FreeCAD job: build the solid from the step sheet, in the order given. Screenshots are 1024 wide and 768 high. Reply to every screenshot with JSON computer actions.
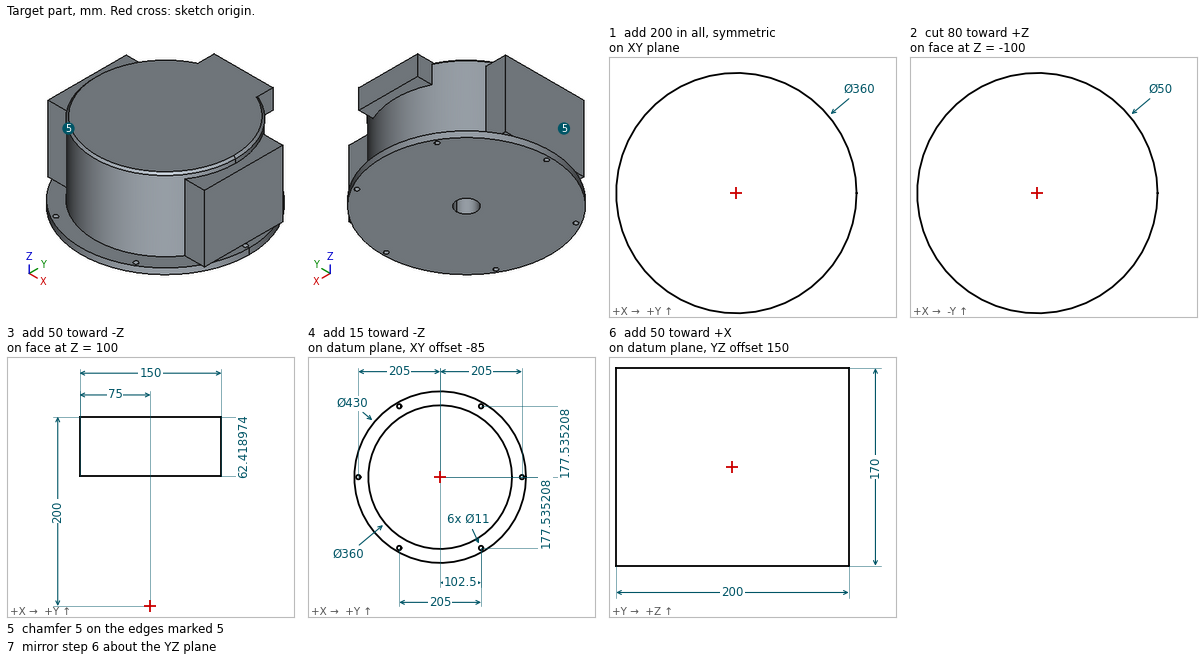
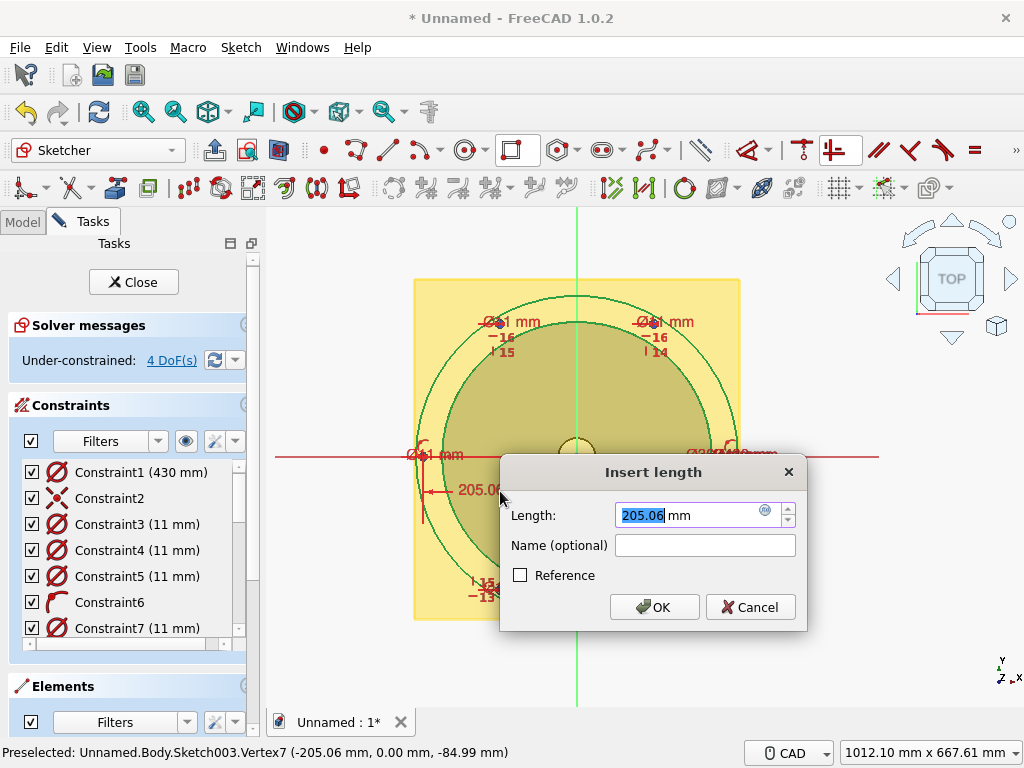
{"action": "type", "text": "205"}
{"action": "key", "text": "Return"}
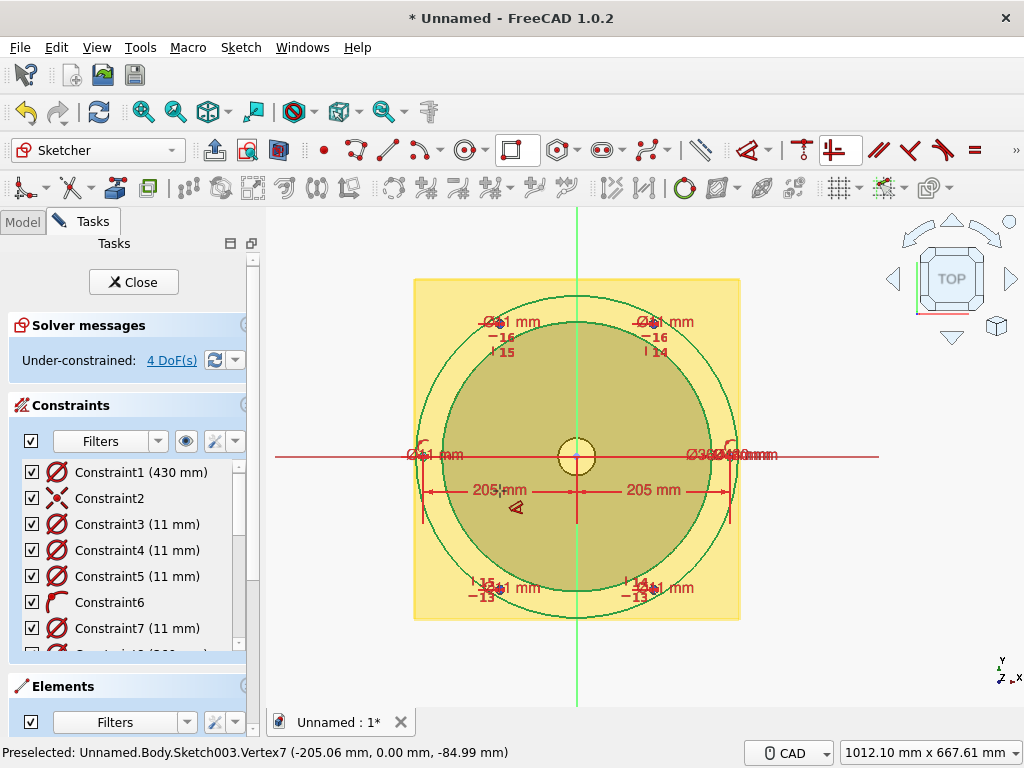
{"action": "left_click", "coordinate": [654, 590]}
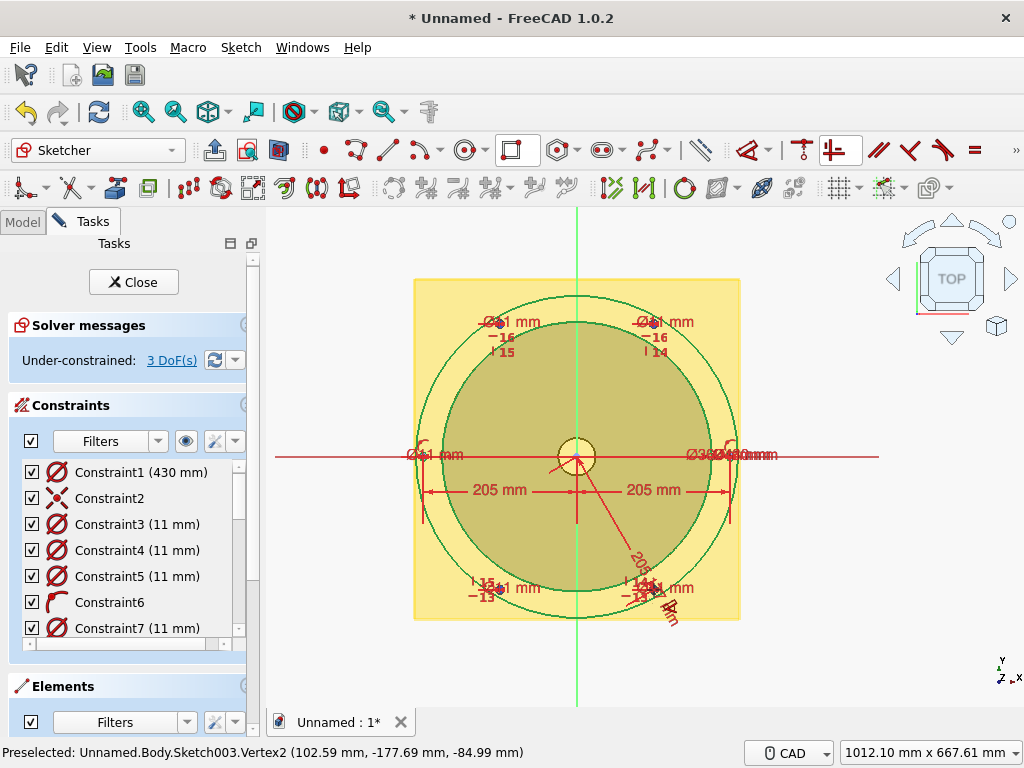
{"action": "left_click", "coordinate": [500, 590]}
{"action": "left_click", "coordinate": [523, 624]}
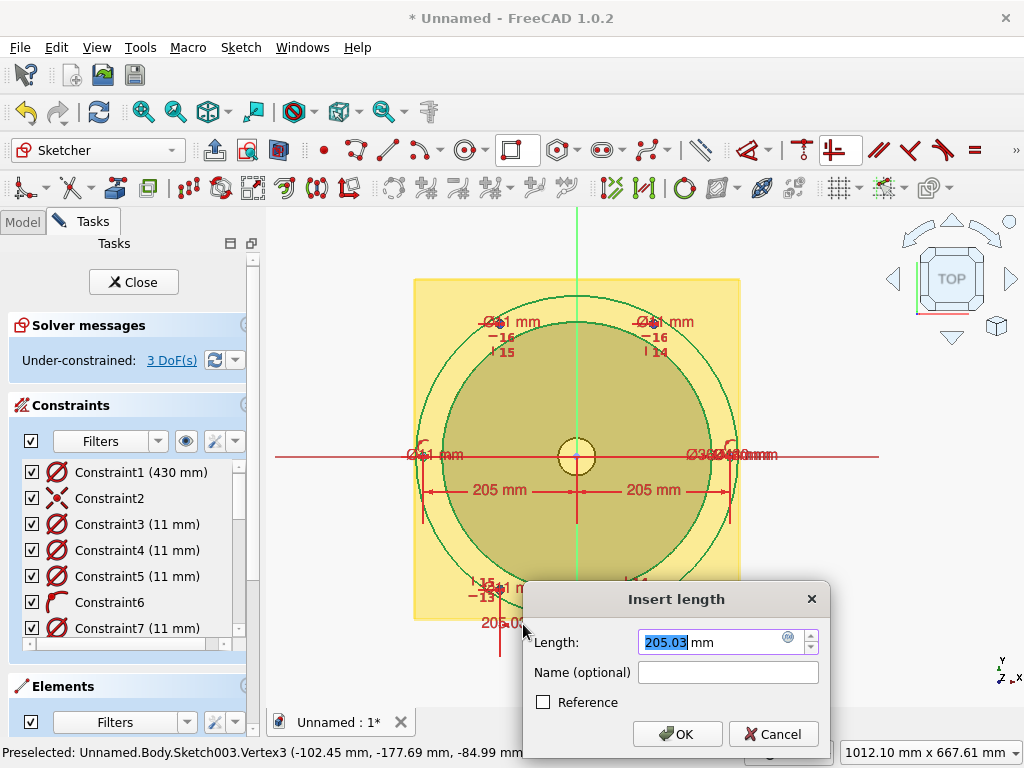
{"action": "type", "text": "205"}
{"action": "key", "text": "Return"}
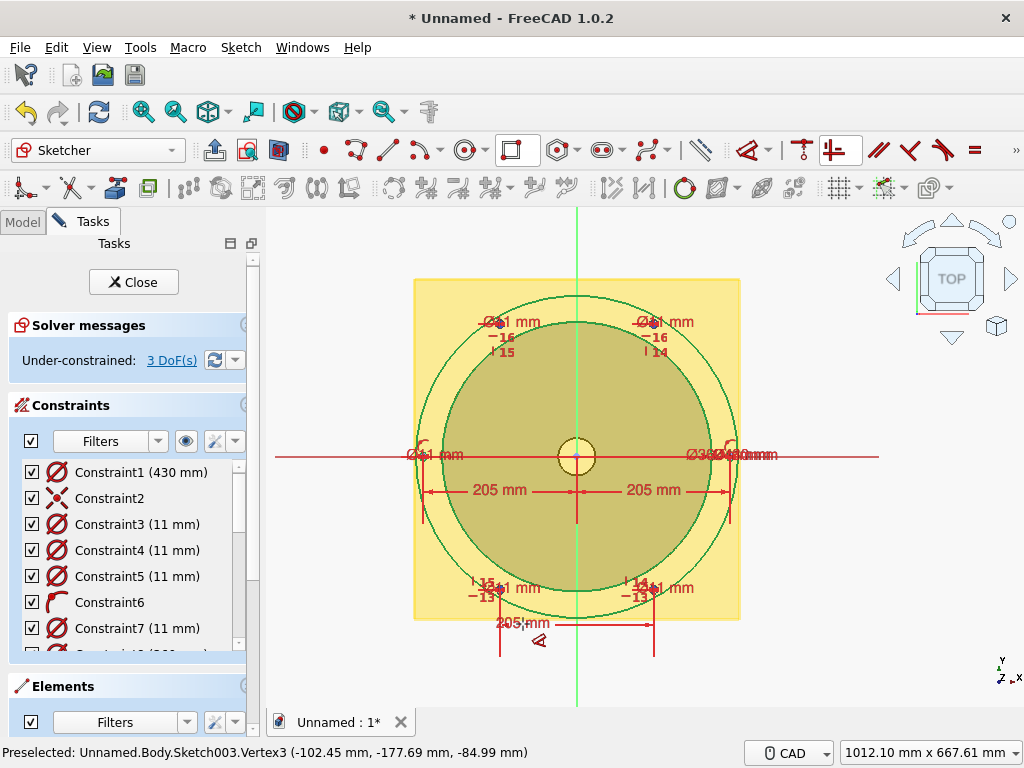
{"action": "left_click", "coordinate": [654, 590]}
{"action": "left_click", "coordinate": [633, 624]}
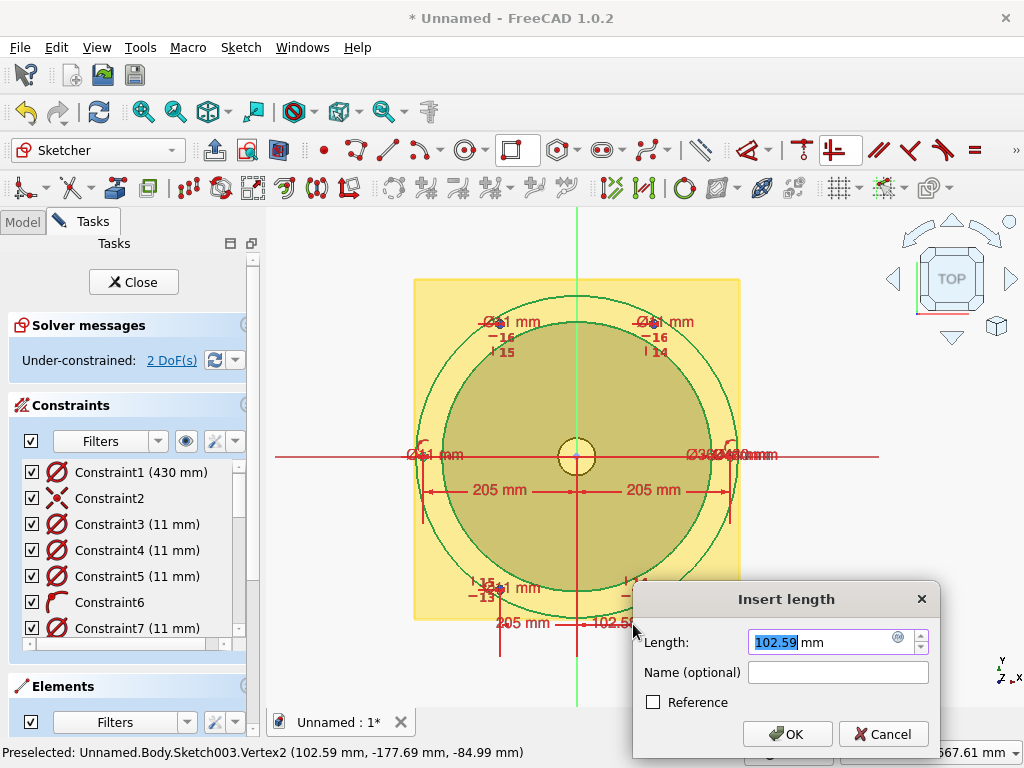
{"action": "type", "text": "102.5"}
{"action": "key", "text": "Return"}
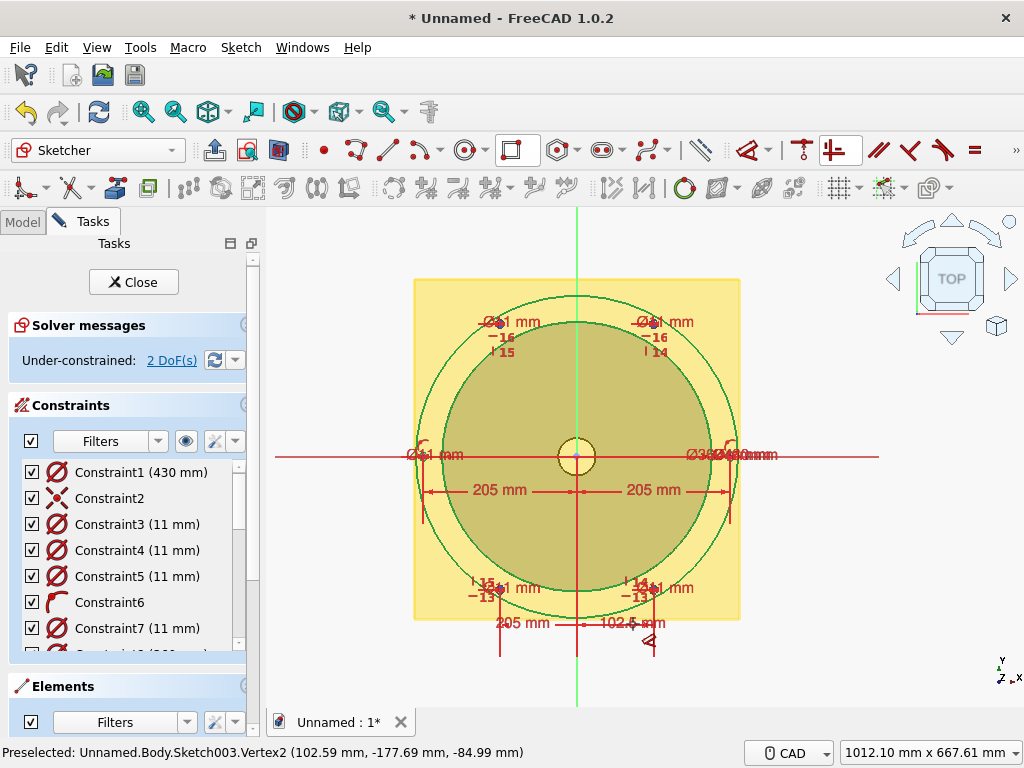
{"action": "left_click", "coordinate": [654, 590]}
{"action": "left_click", "coordinate": [543, 523]}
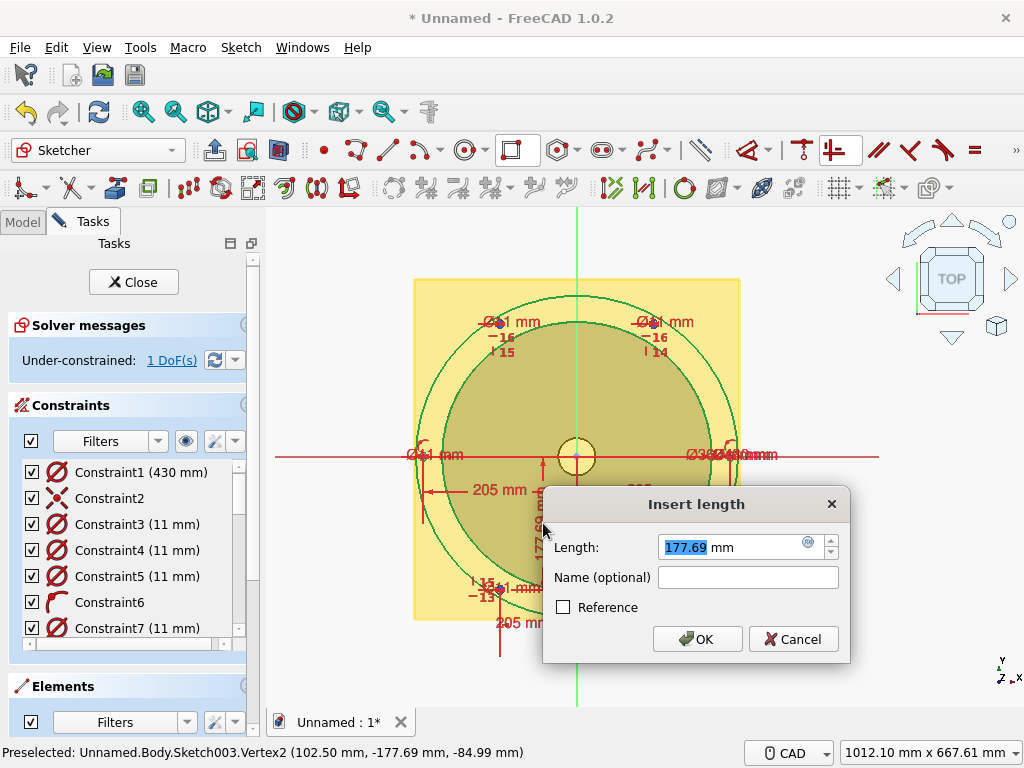
{"action": "type", "text": "177.535208"}
{"action": "key", "text": "Return"}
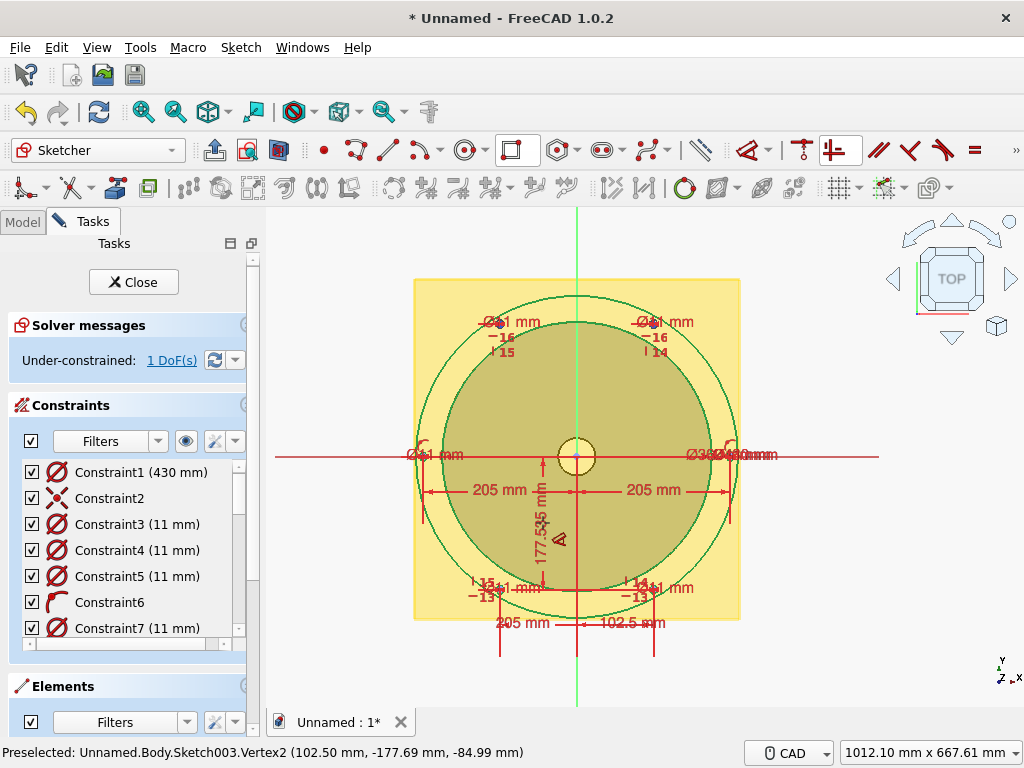
{"action": "left_click", "coordinate": [654, 324]}
{"action": "left_click", "coordinate": [688, 421]}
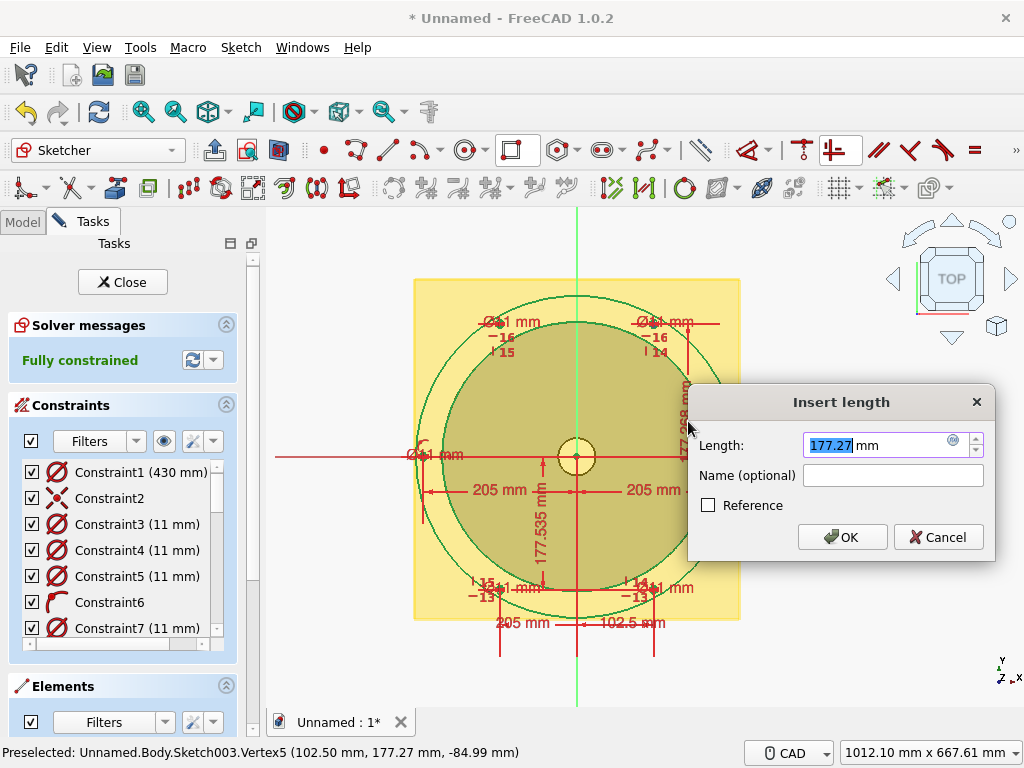
{"action": "type", "text": "177.535208"}
{"action": "key", "text": "Return"}
{"action": "key", "text": "Escape"}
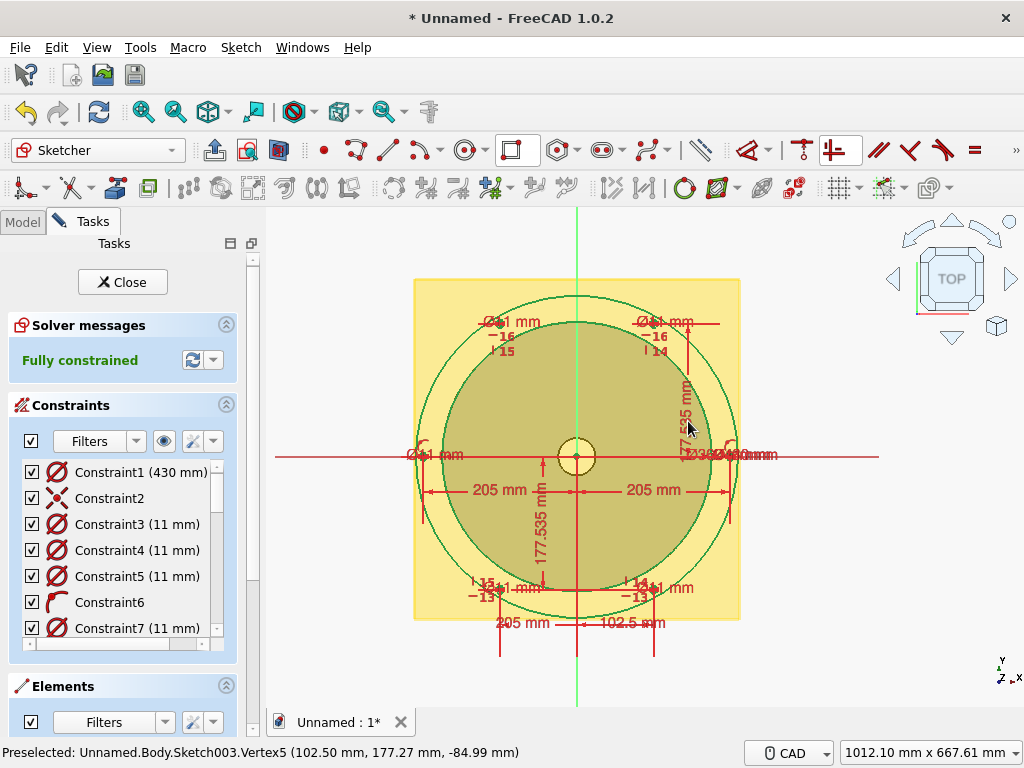
{"action": "left_click", "coordinate": [123, 282]}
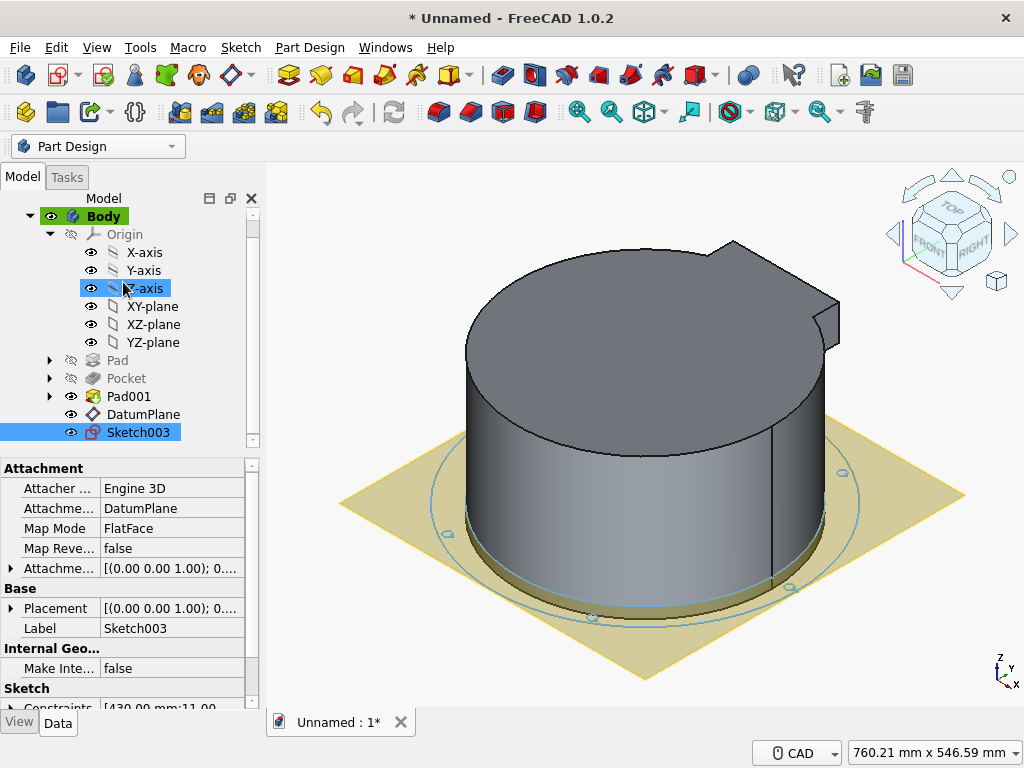
{"action": "left_click", "coordinate": [290, 76]}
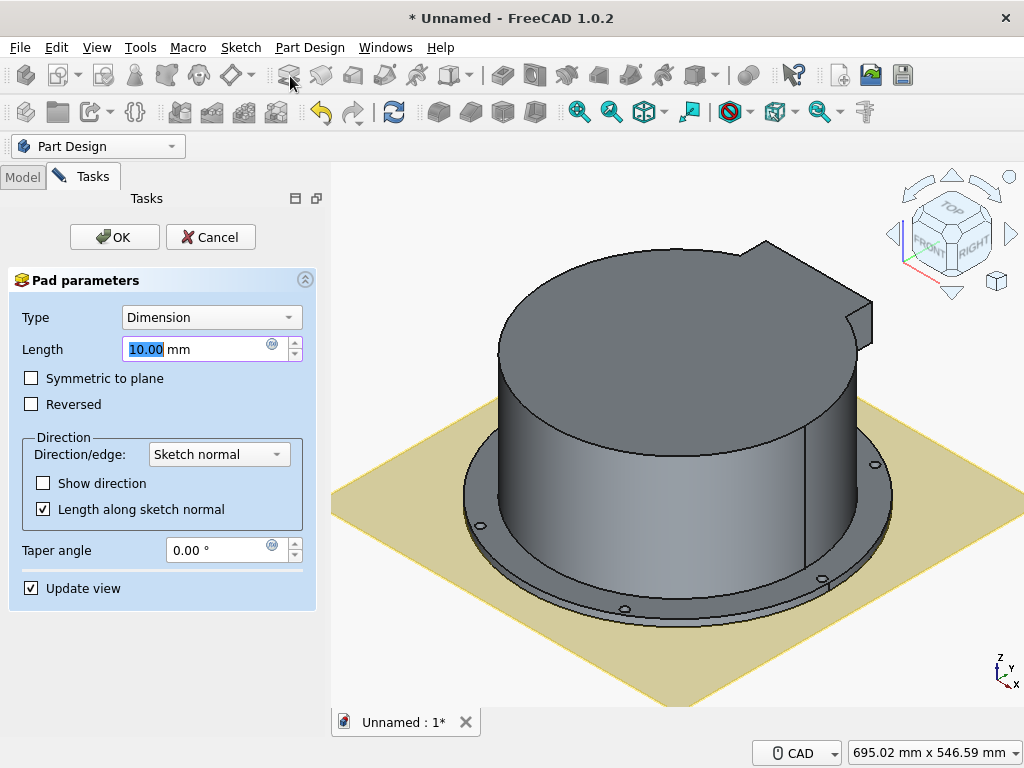
{"action": "type", "text": "15"}
{"action": "key", "text": "Tab"}